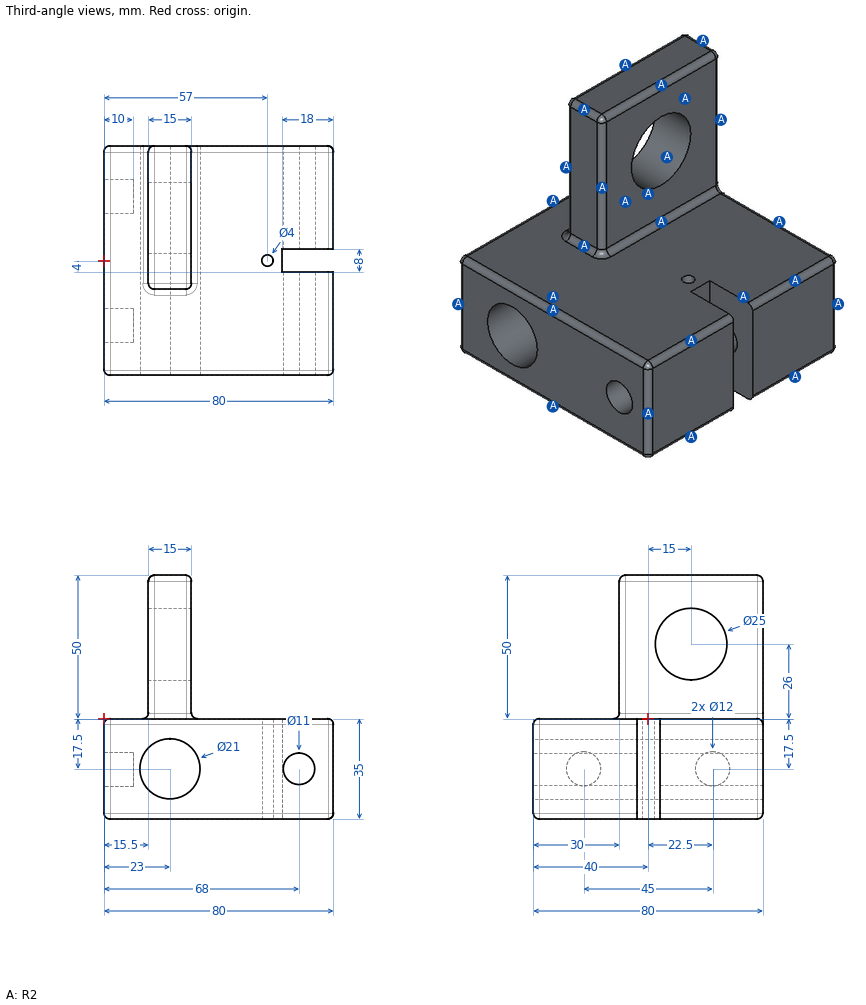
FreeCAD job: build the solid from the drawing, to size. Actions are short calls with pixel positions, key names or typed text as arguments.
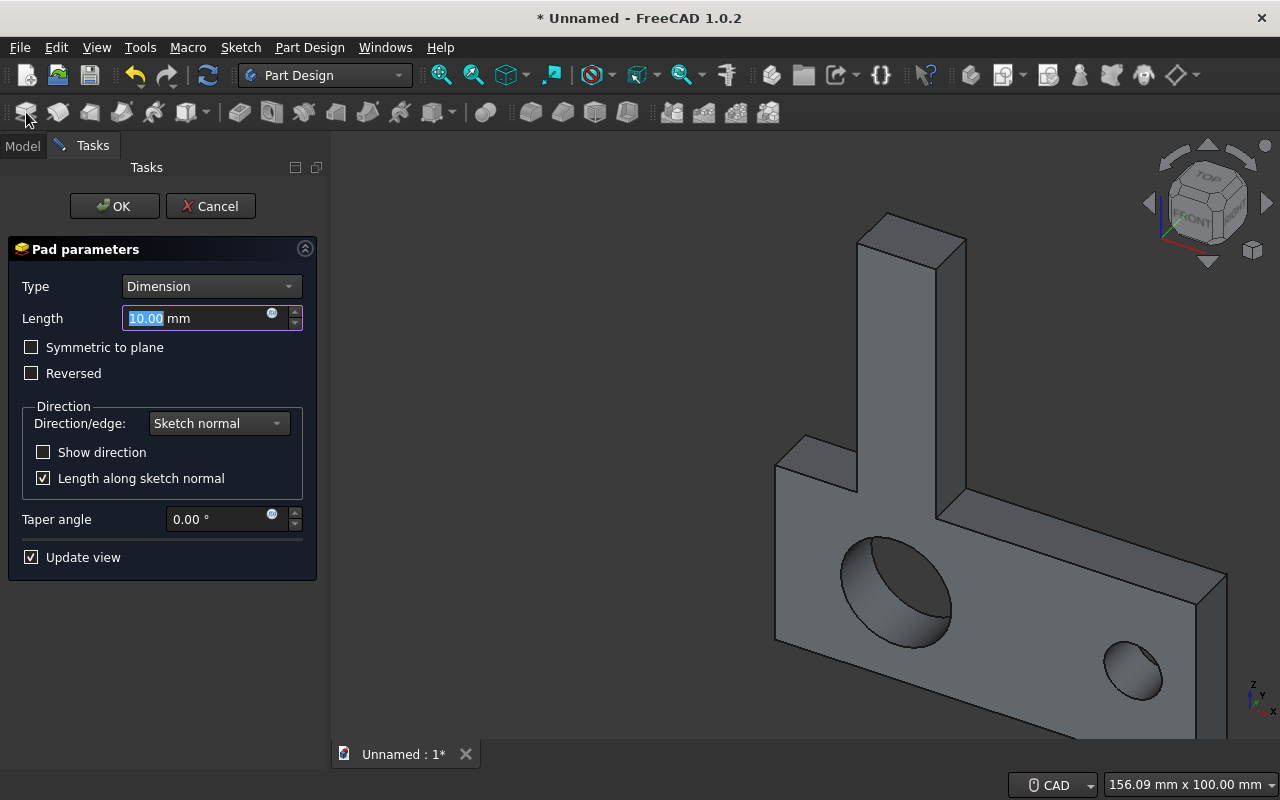
text(80)
key(Tab)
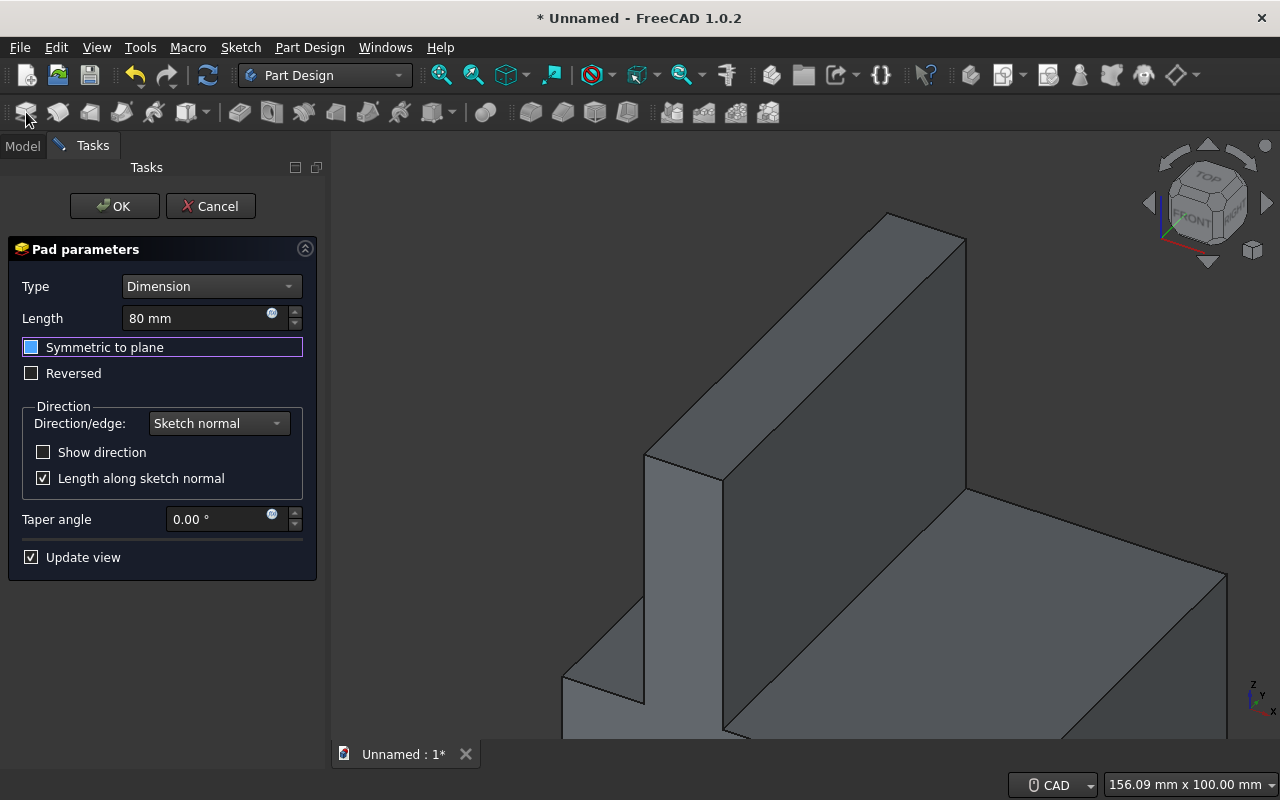
click(30, 347)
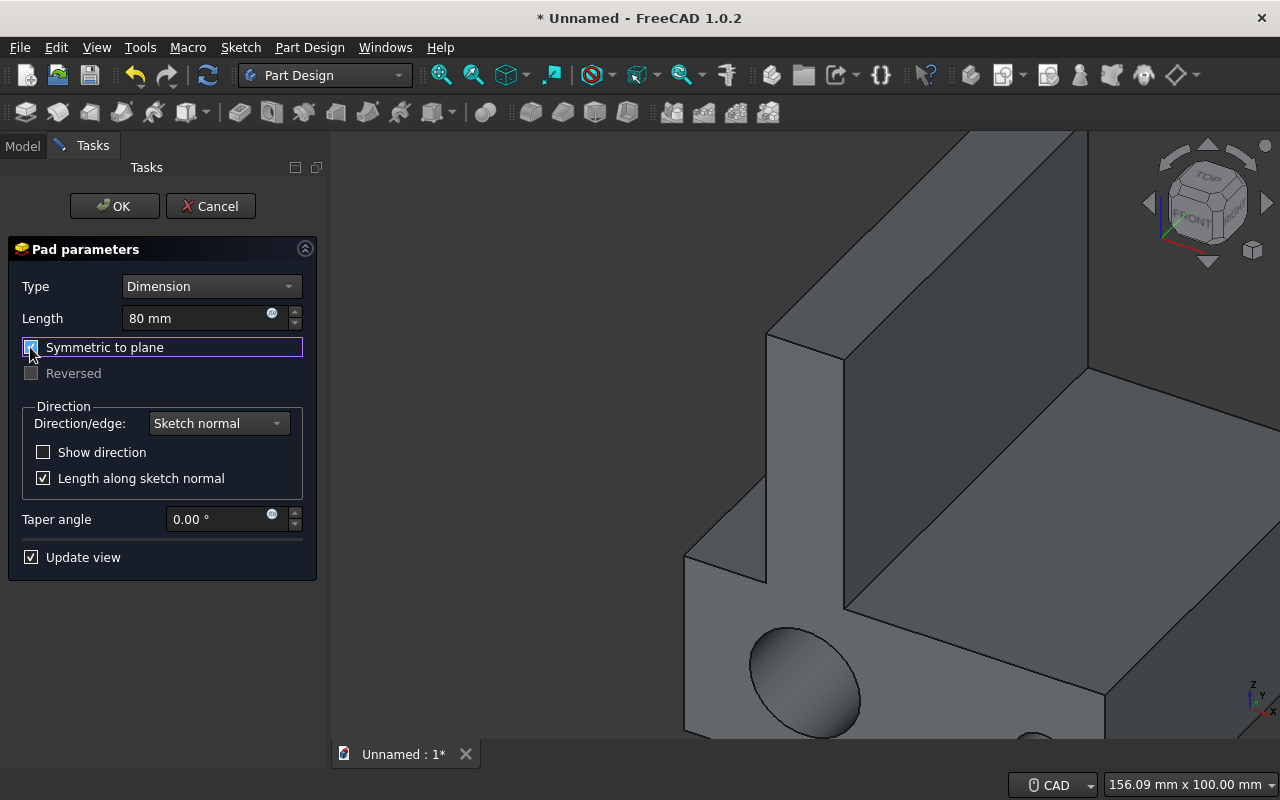
click(115, 206)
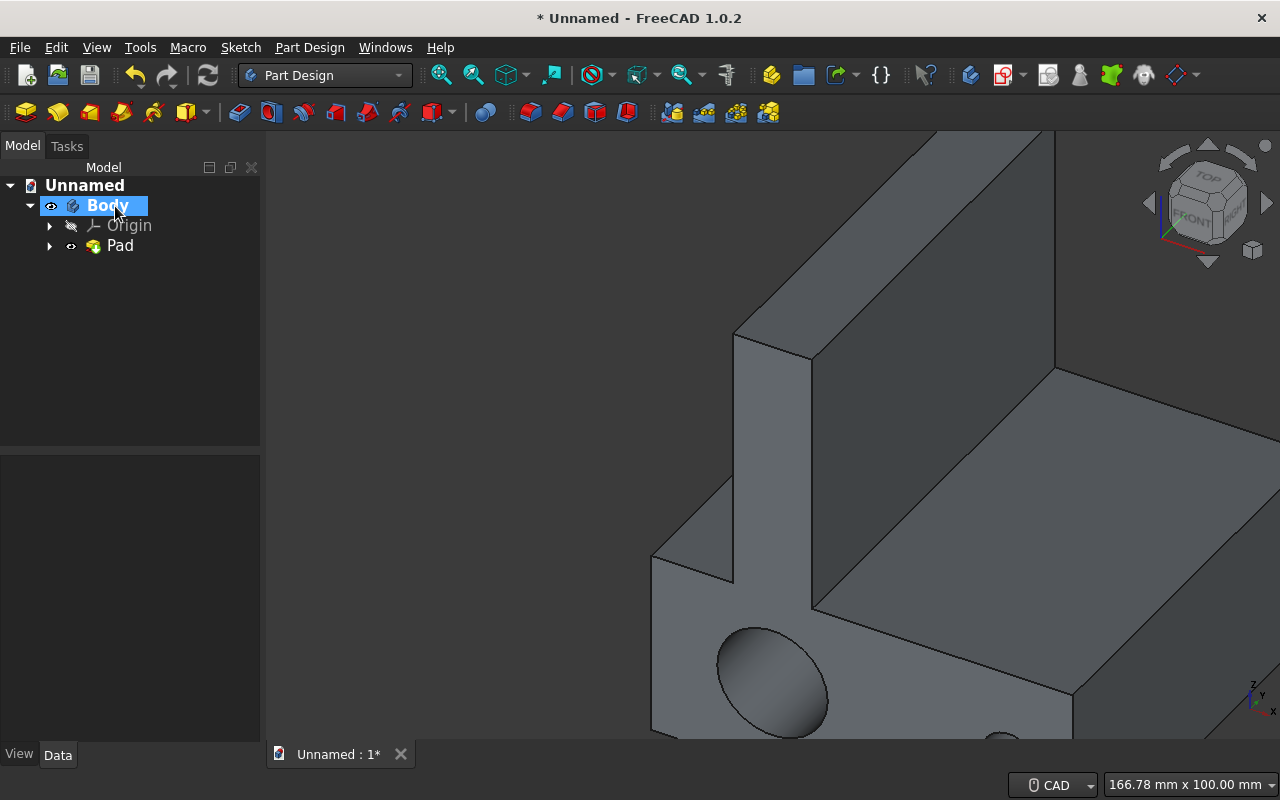
click(442, 76)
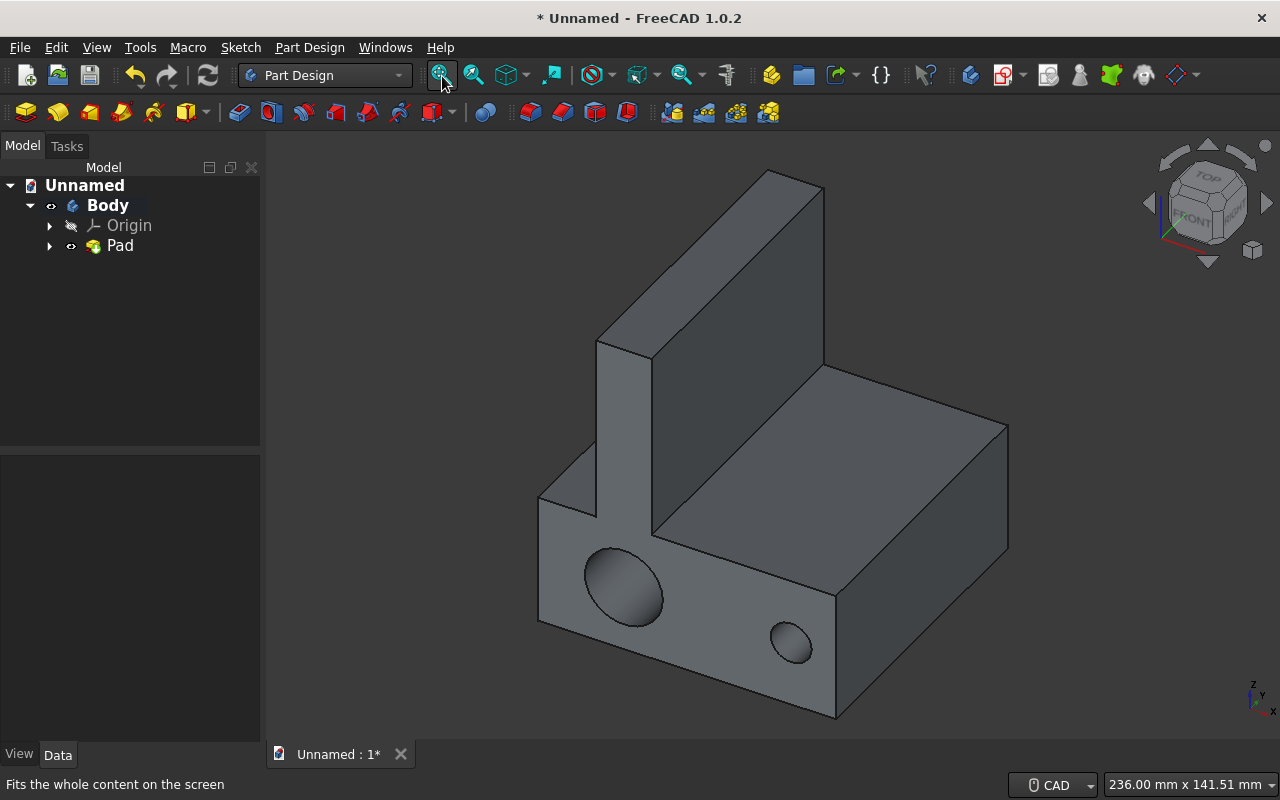
click(1004, 76)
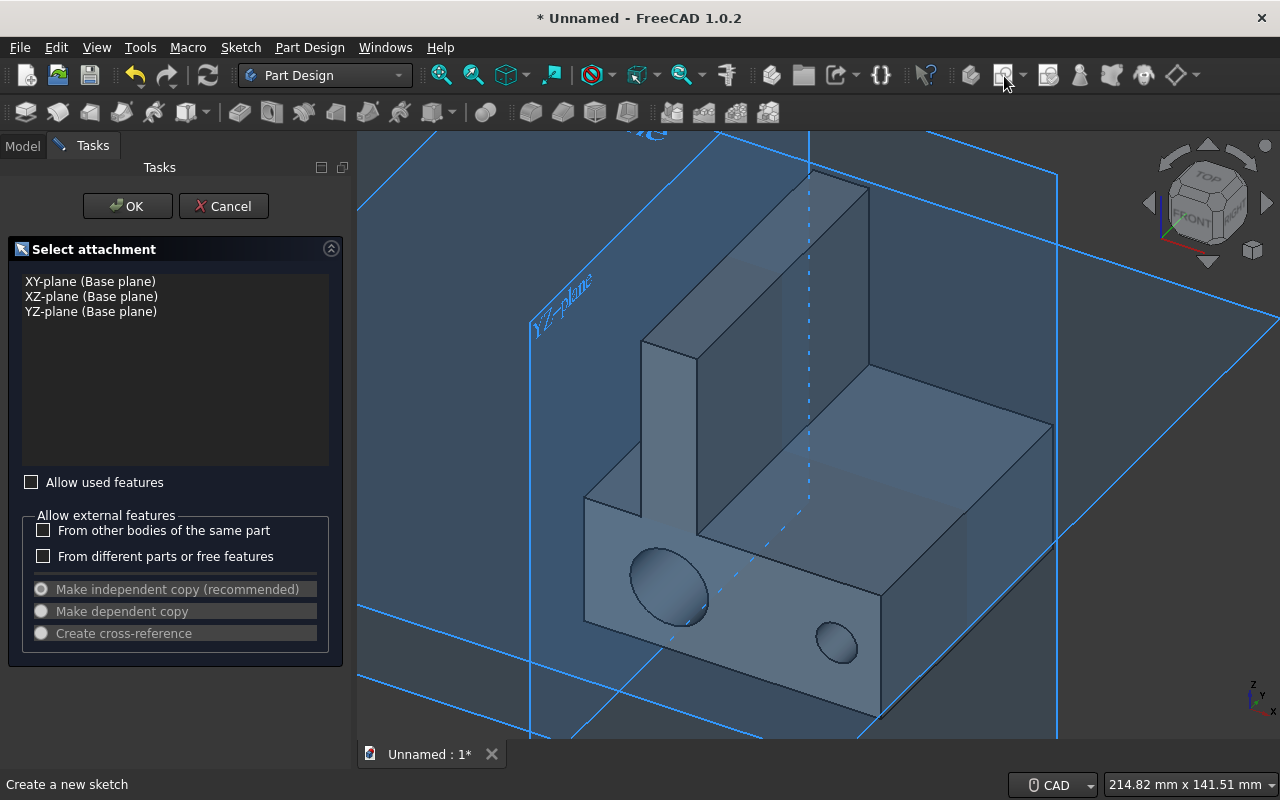
click(82, 312)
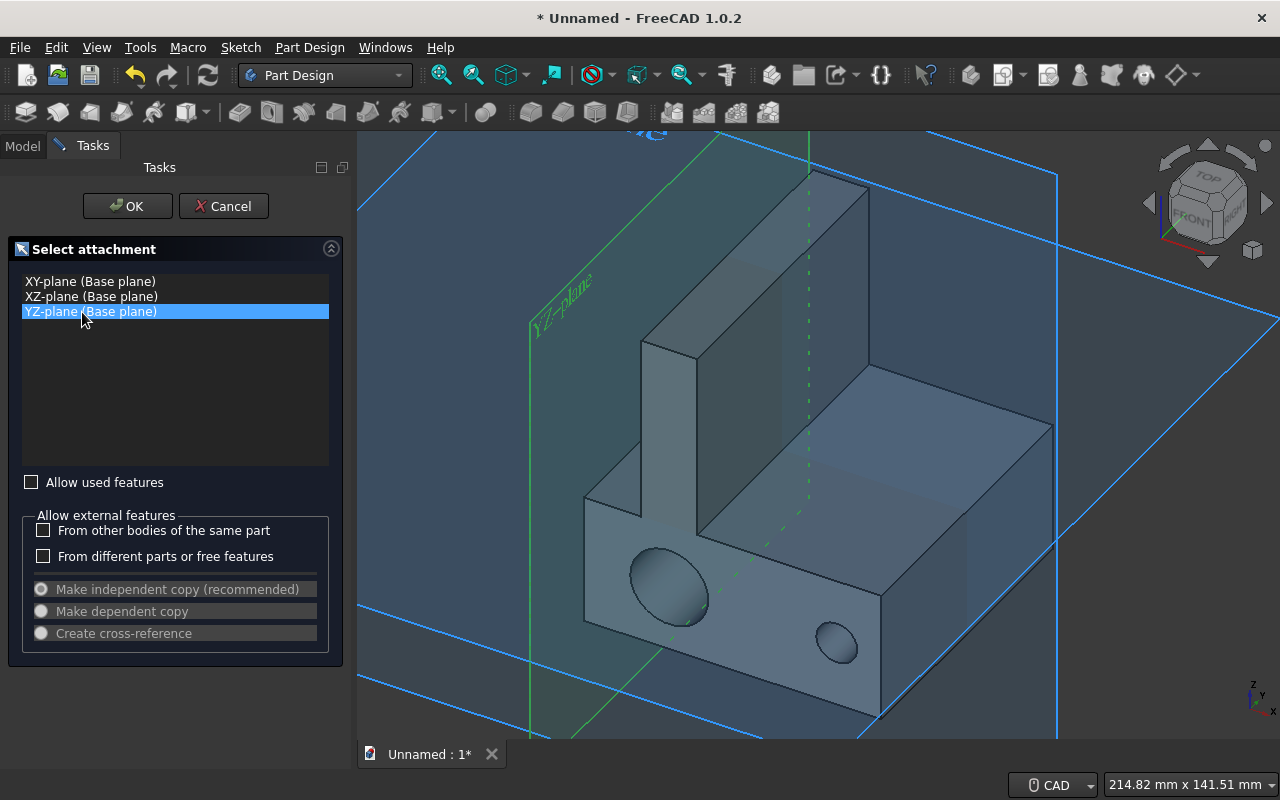
click(128, 206)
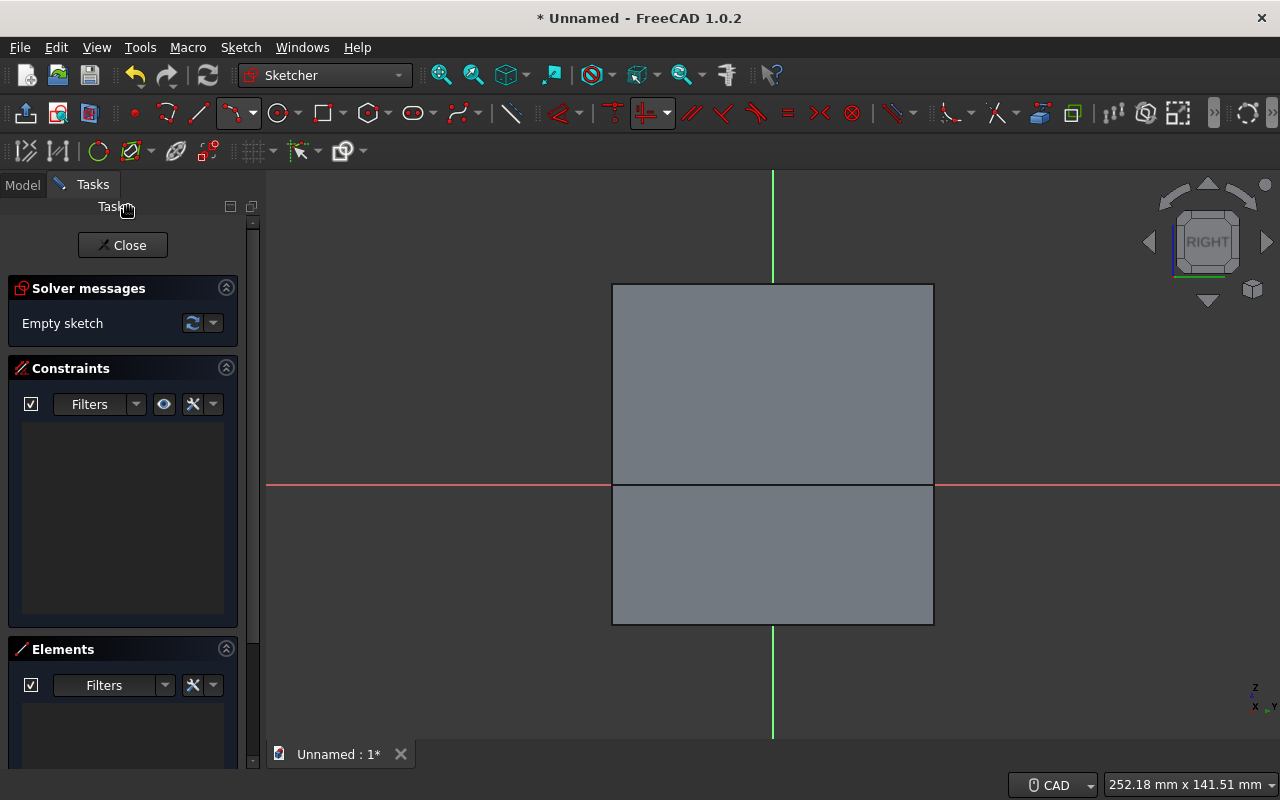
click(90, 114)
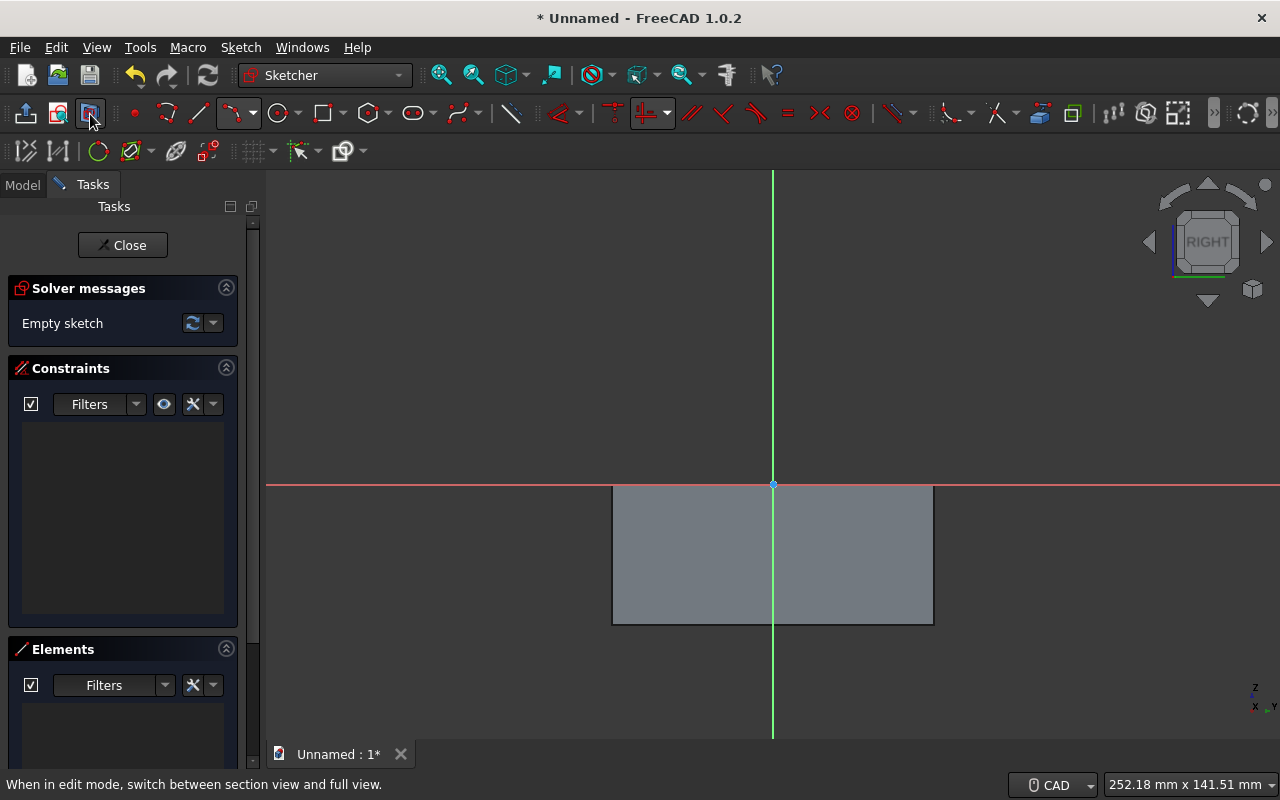
scroll(813, 577, up, 5)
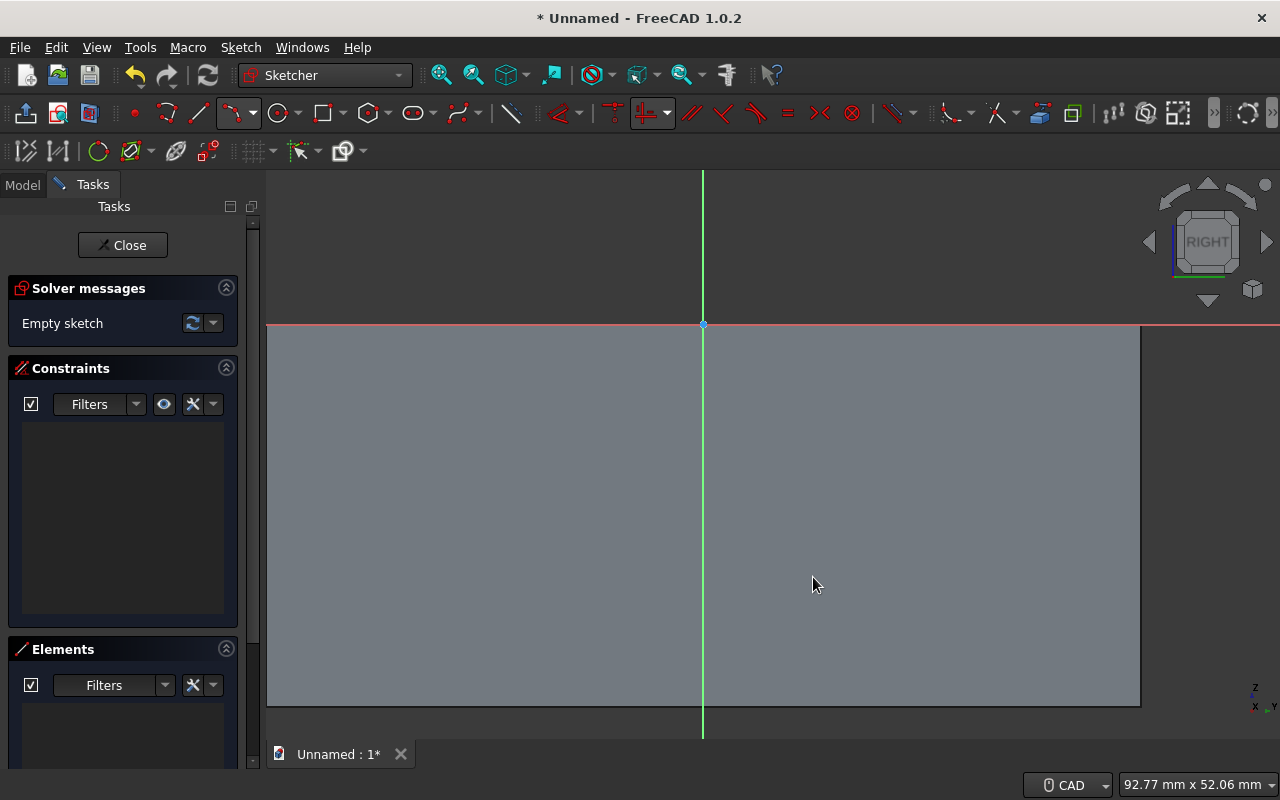
click(278, 114)